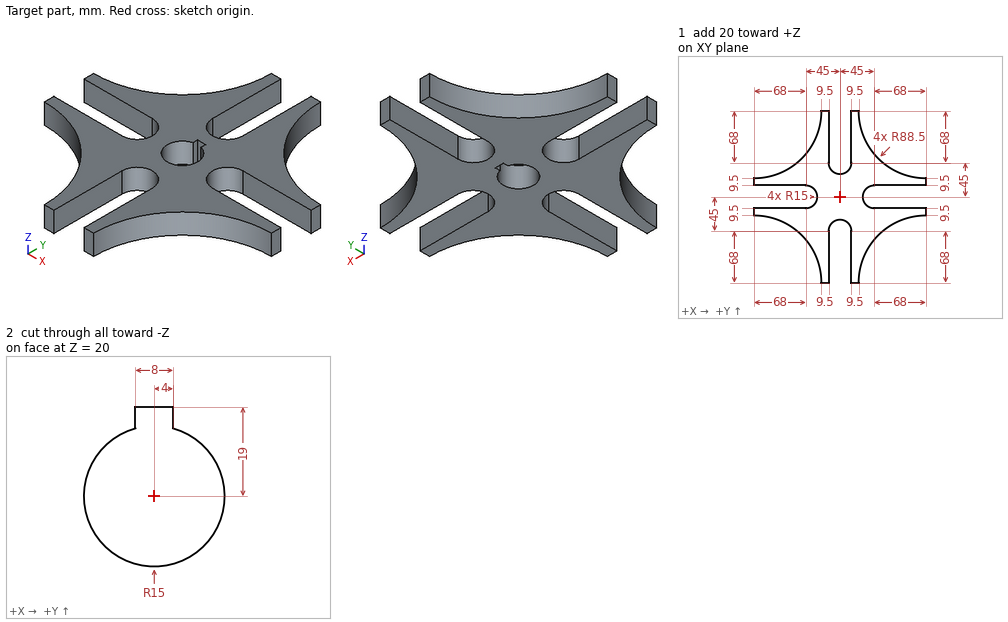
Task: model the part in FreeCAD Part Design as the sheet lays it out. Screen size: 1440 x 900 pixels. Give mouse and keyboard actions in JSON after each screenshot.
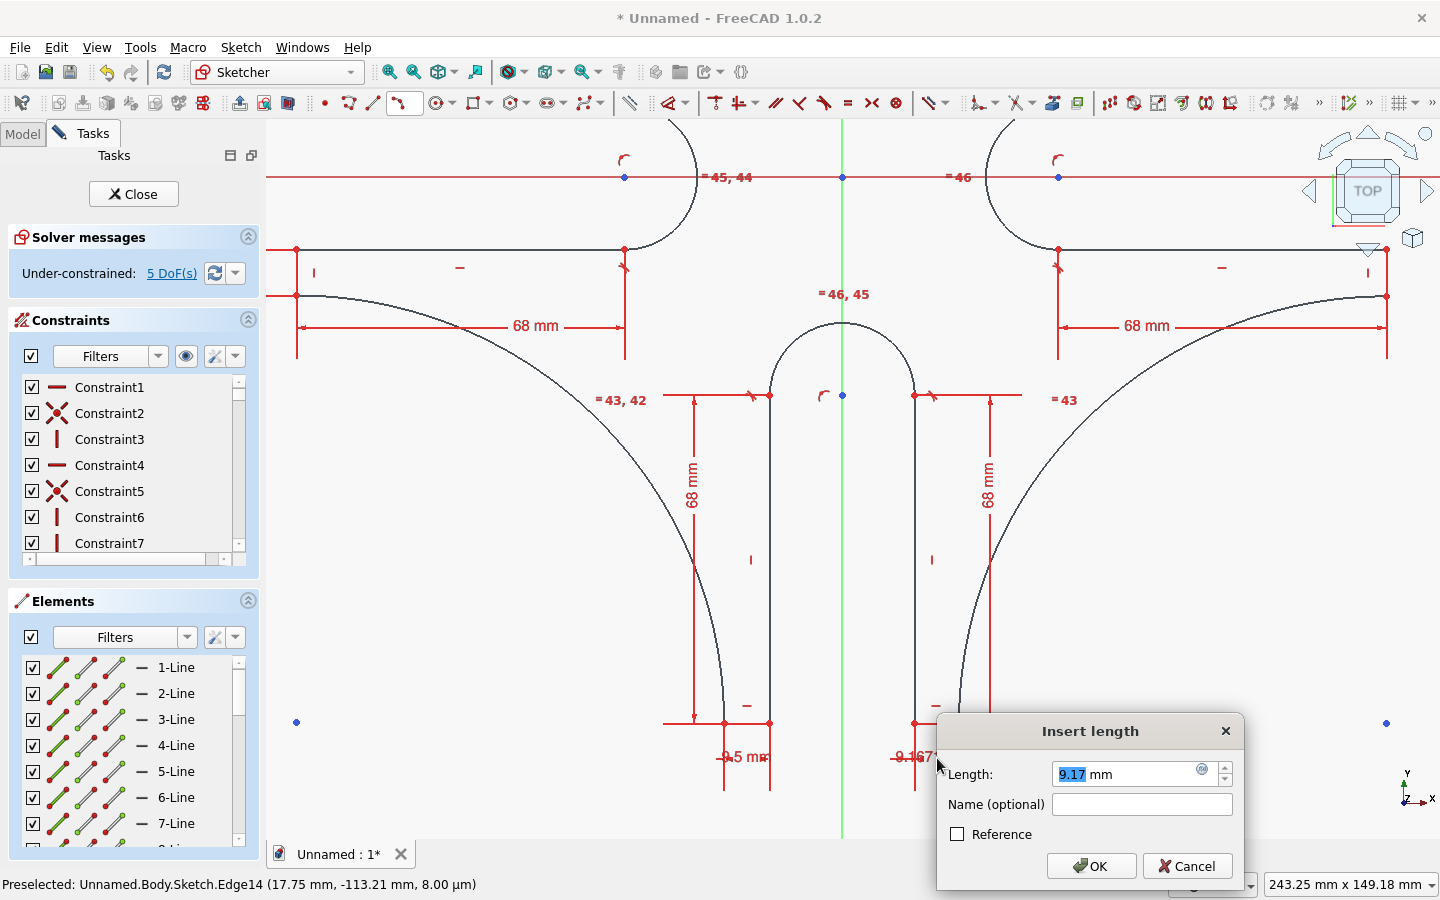
{"action": "type", "text": "9.5"}
{"action": "key", "text": "Return"}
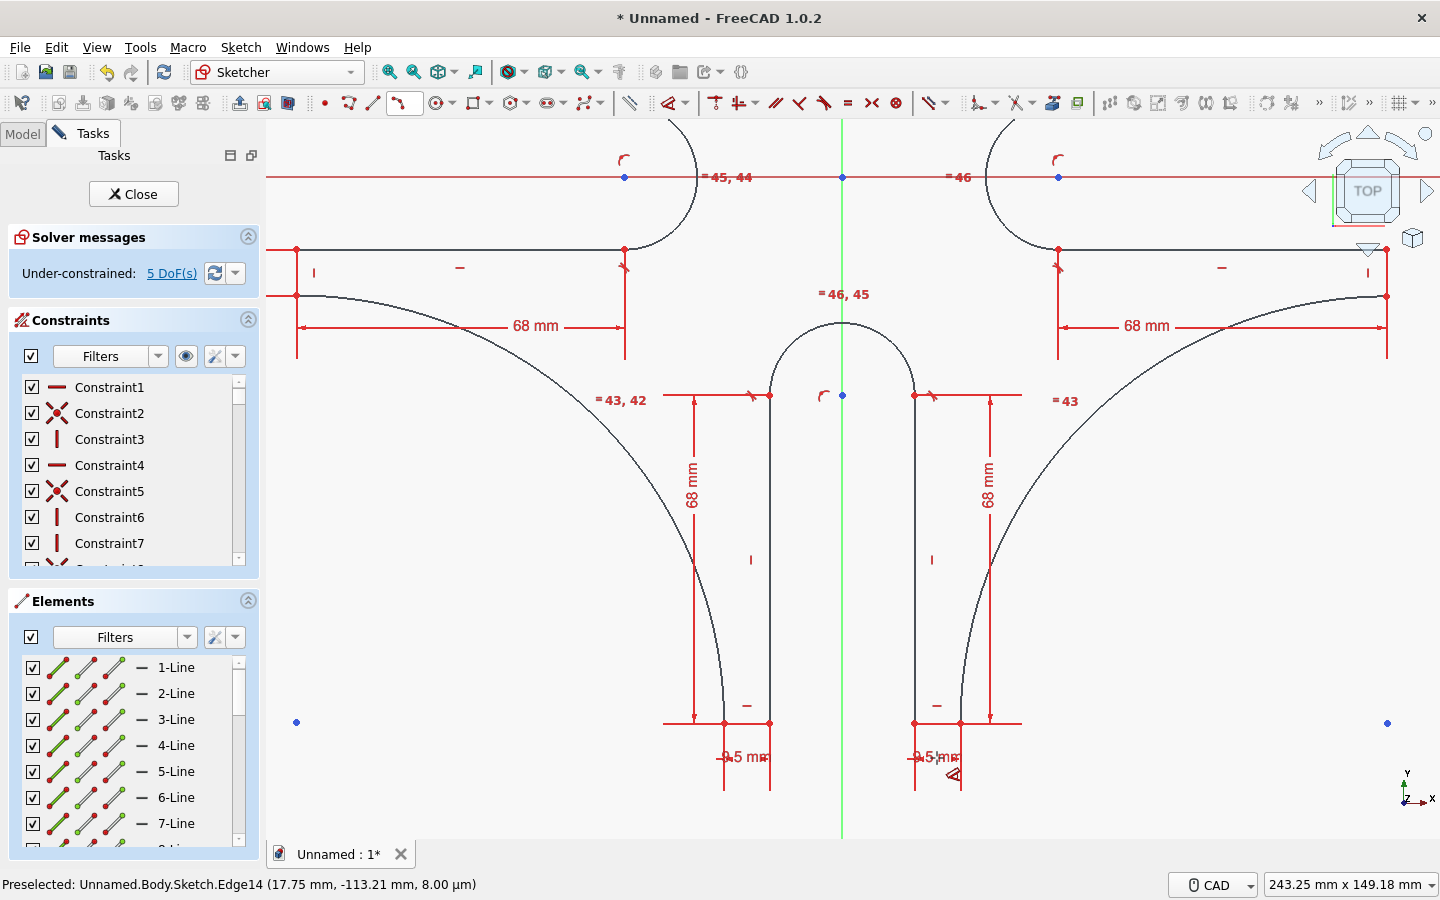
{"action": "scroll", "coordinate": [737, 725], "scroll_direction": "down", "scroll_amount": 4}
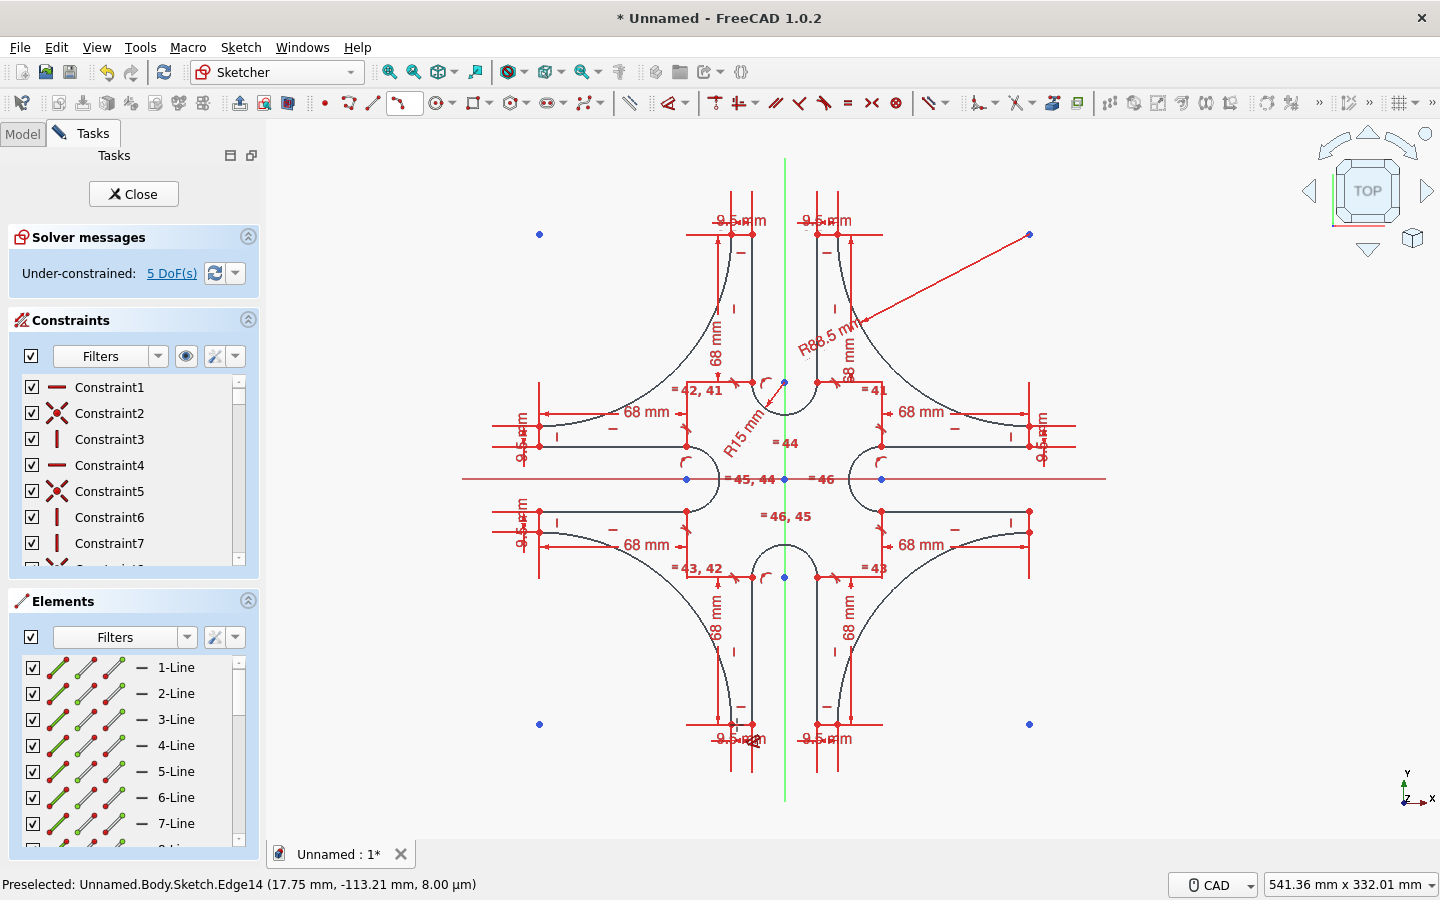
{"action": "scroll", "coordinate": [1029, 527], "scroll_direction": "up", "scroll_amount": 4}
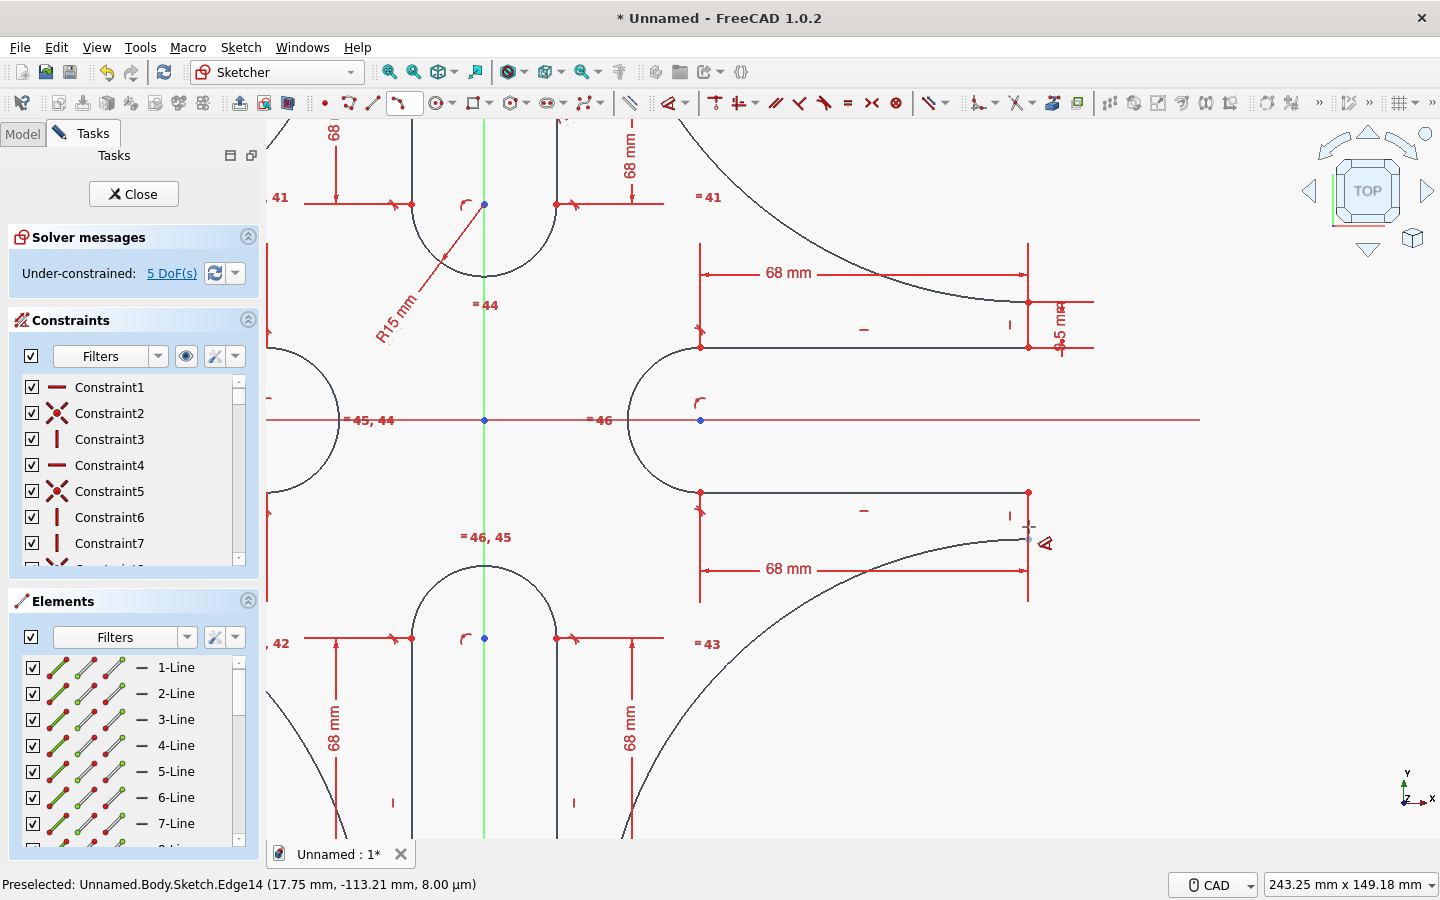
{"action": "left_click", "coordinate": [1028, 525]}
{"action": "left_click", "coordinate": [1062, 516]}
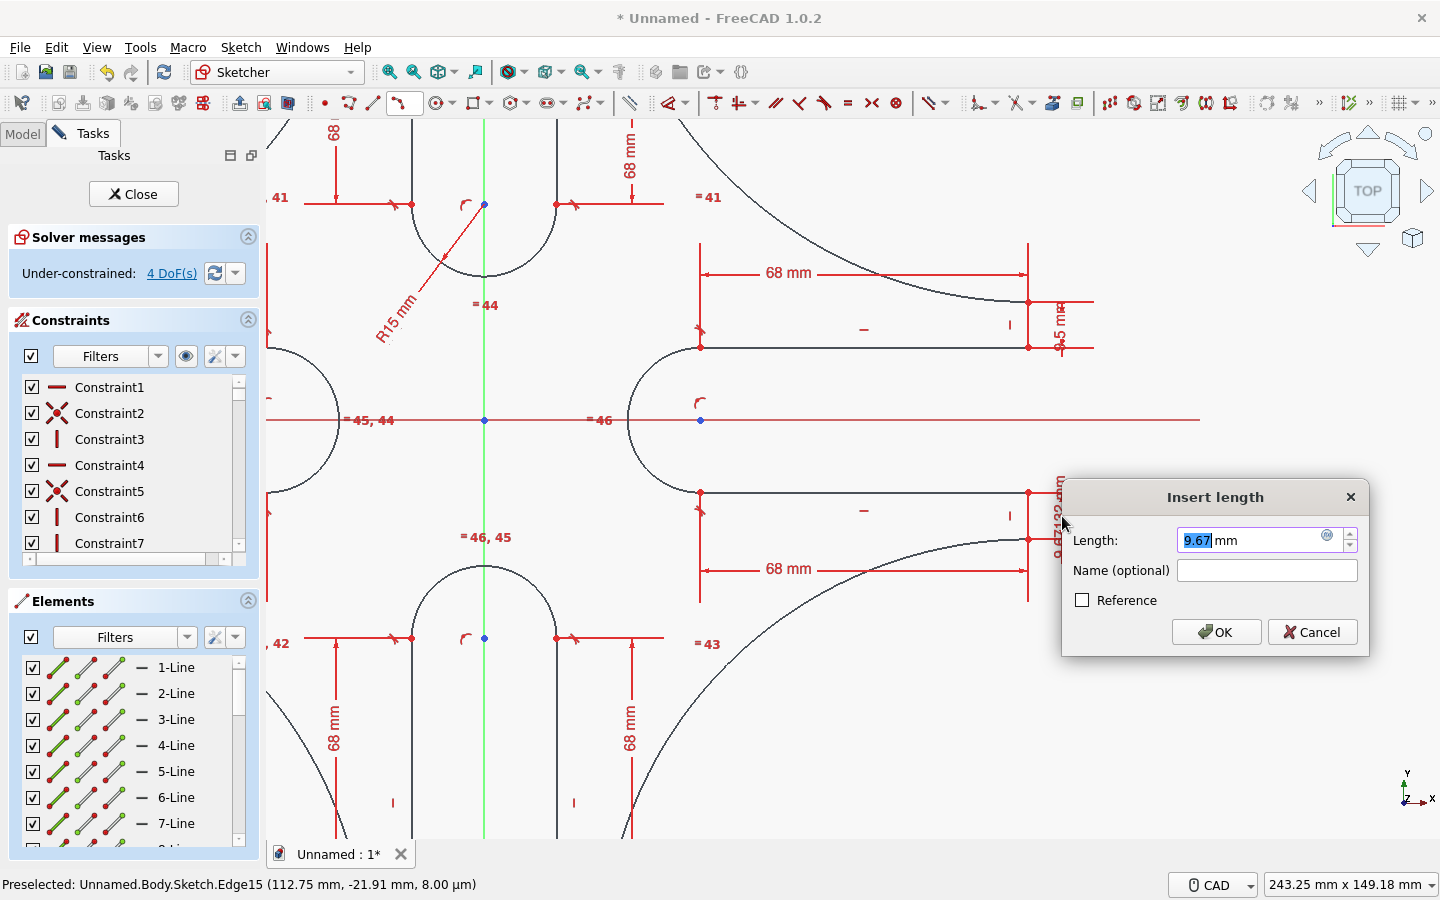
{"action": "type", "text": "9.5"}
{"action": "key", "text": "Return"}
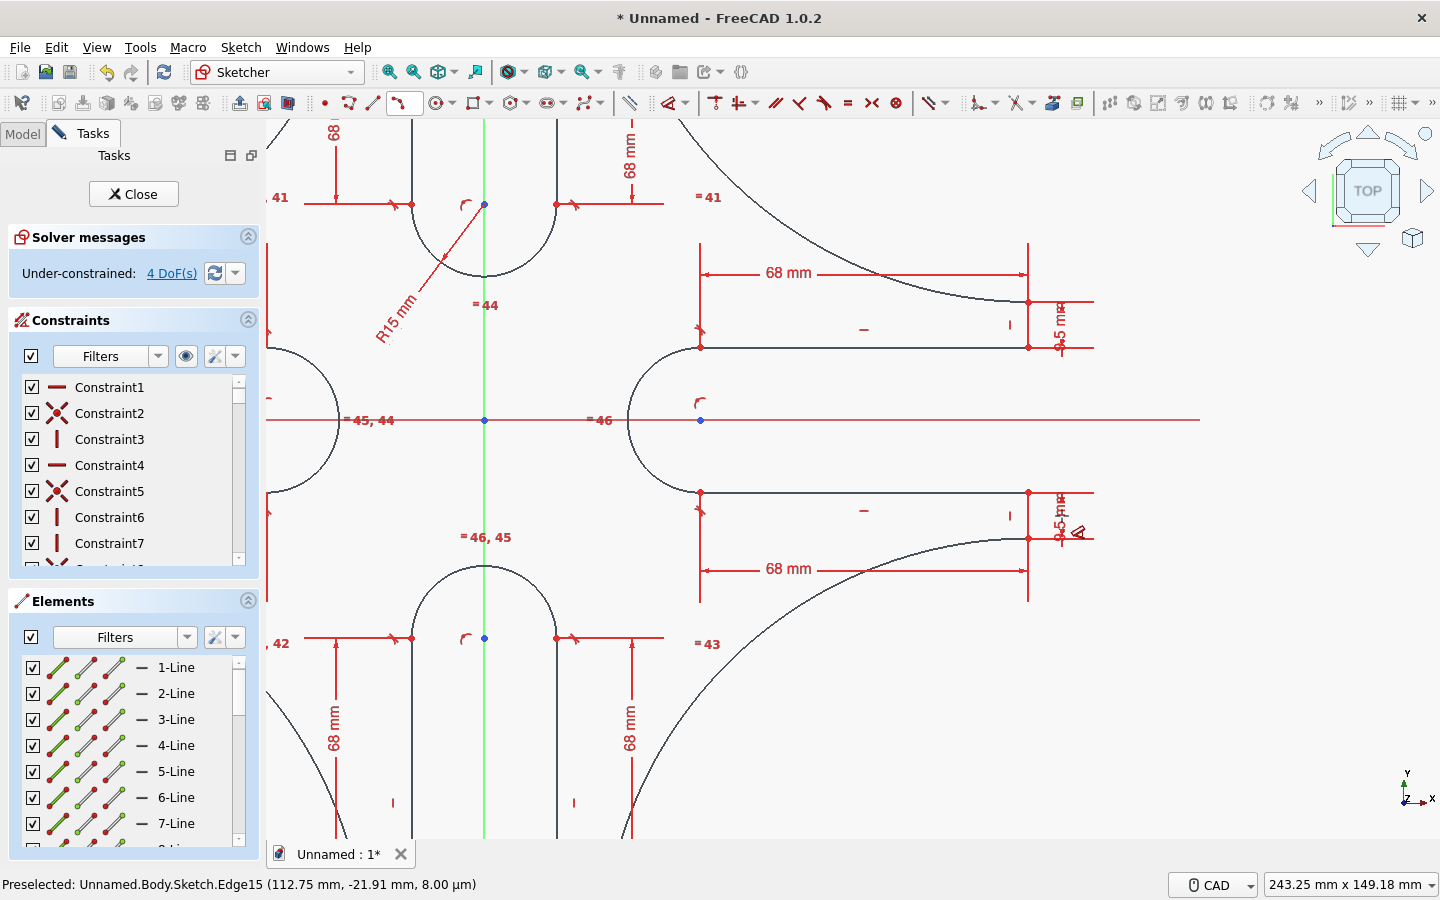
{"action": "left_click", "coordinate": [700, 348]}
{"action": "left_click", "coordinate": [592, 314]}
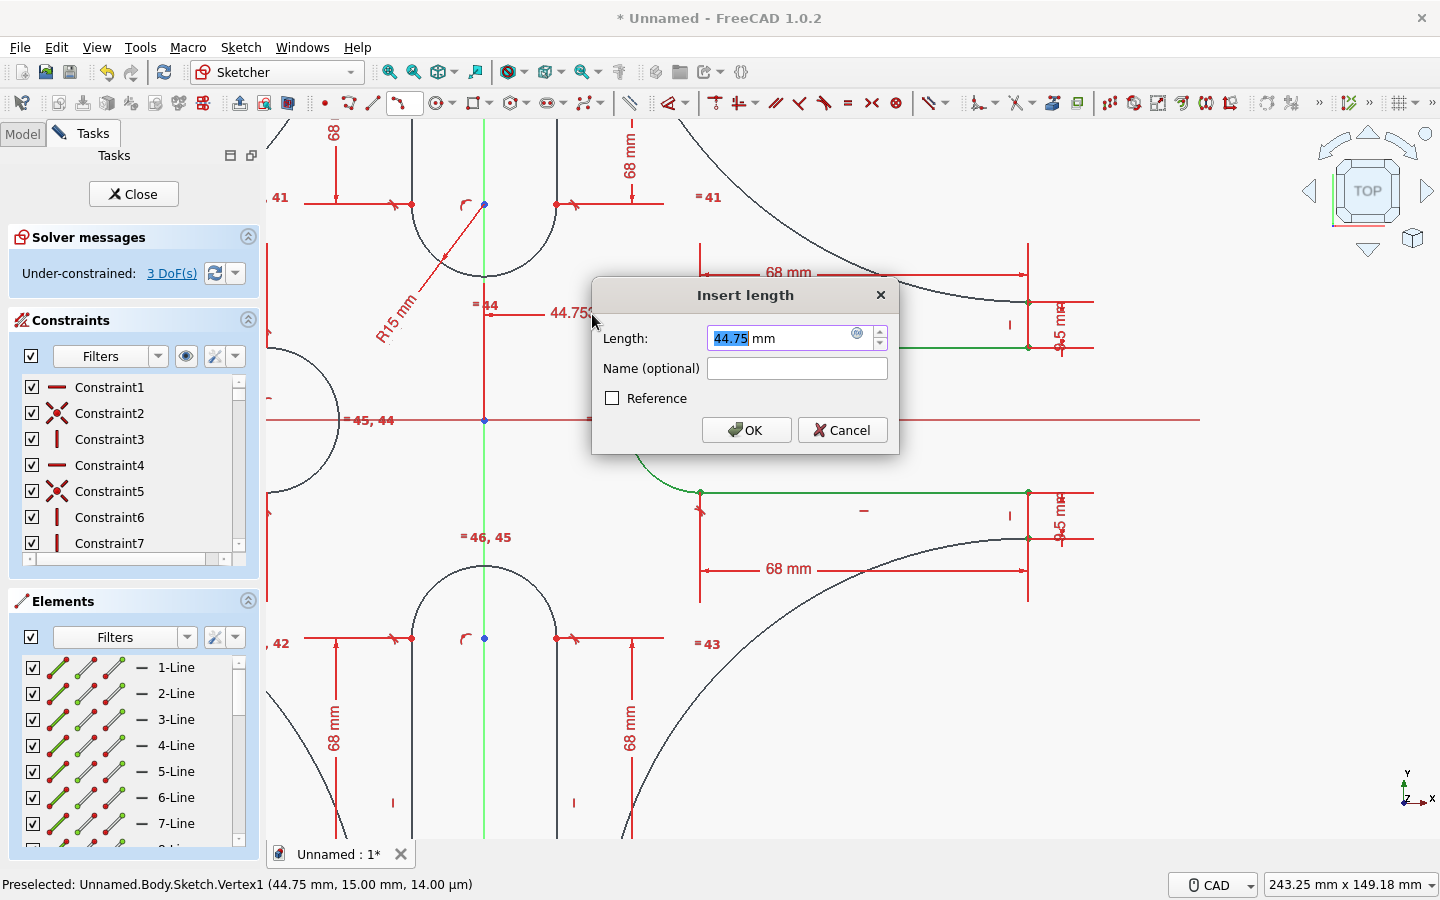
{"action": "type", "text": "45"}
{"action": "key", "text": "Return"}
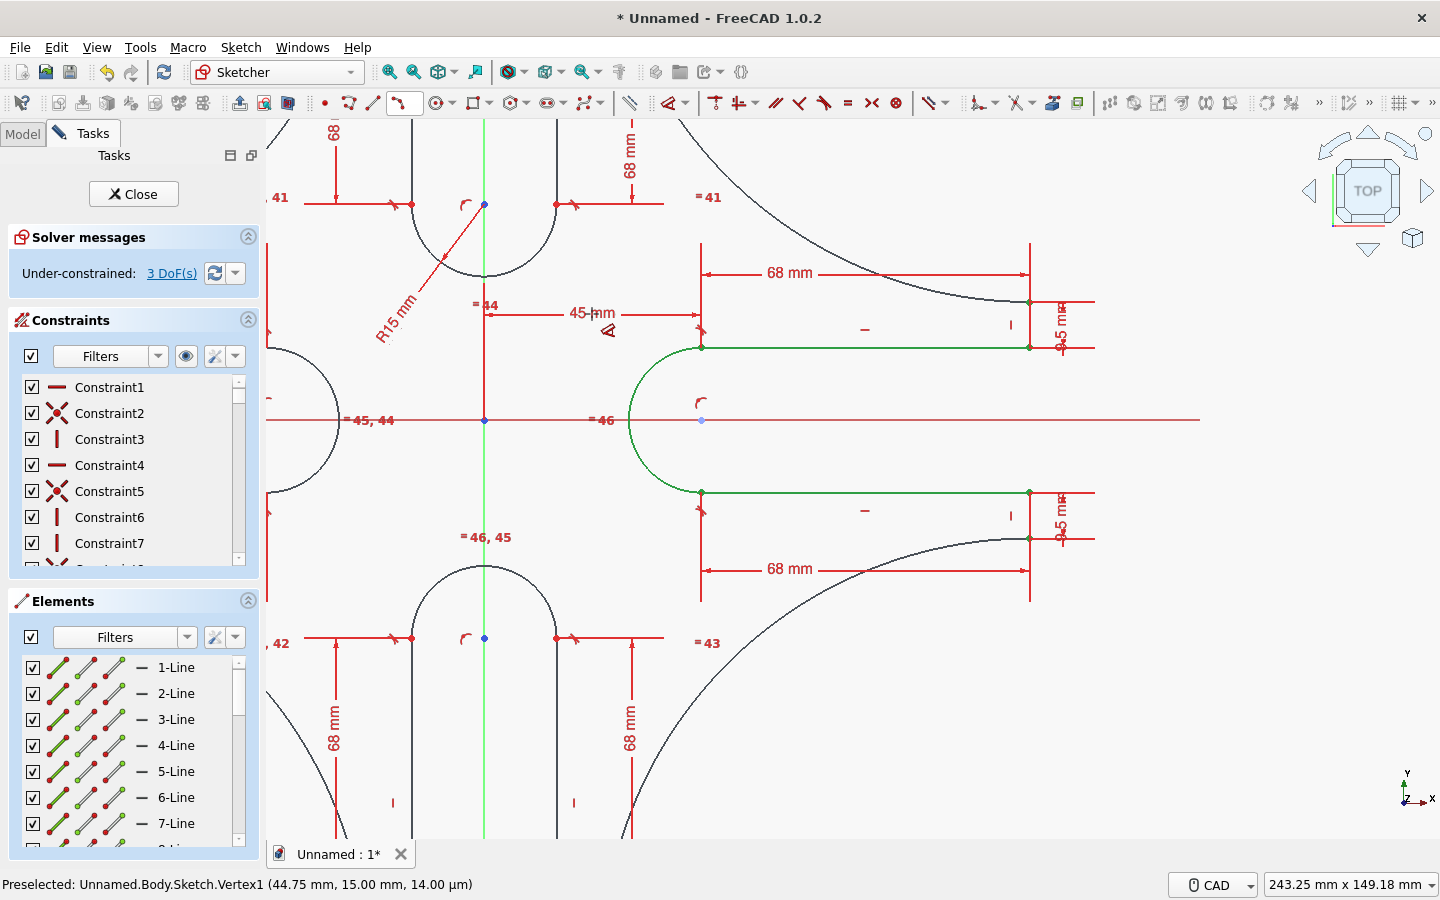
{"action": "left_click", "coordinate": [557, 204]}
{"action": "left_click", "coordinate": [591, 263]}